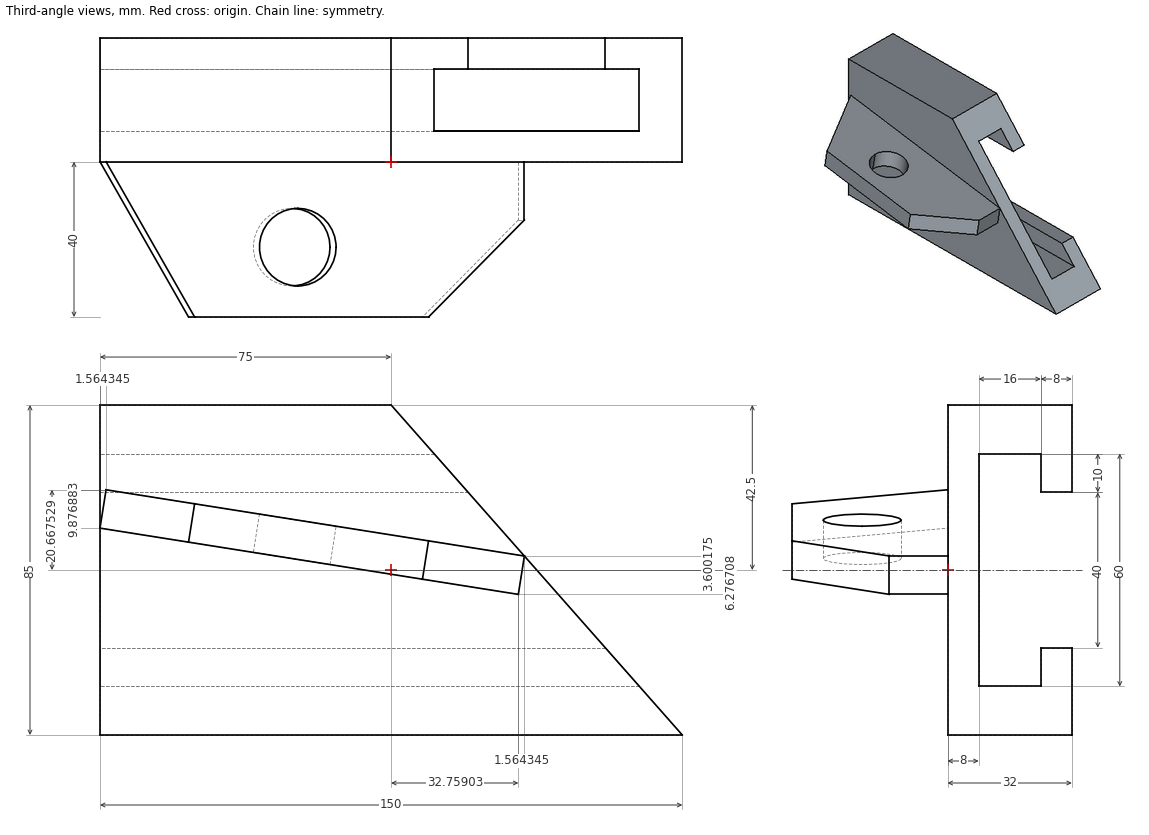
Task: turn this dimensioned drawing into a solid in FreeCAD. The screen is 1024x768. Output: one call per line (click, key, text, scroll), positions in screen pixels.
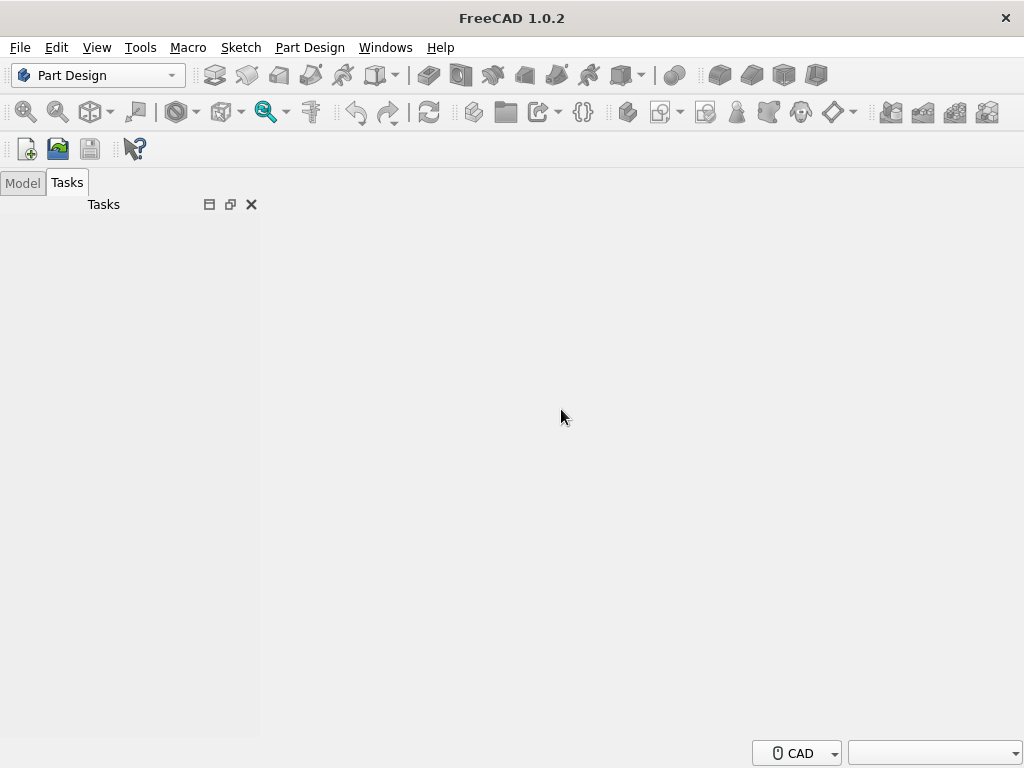
key(ctrl+n)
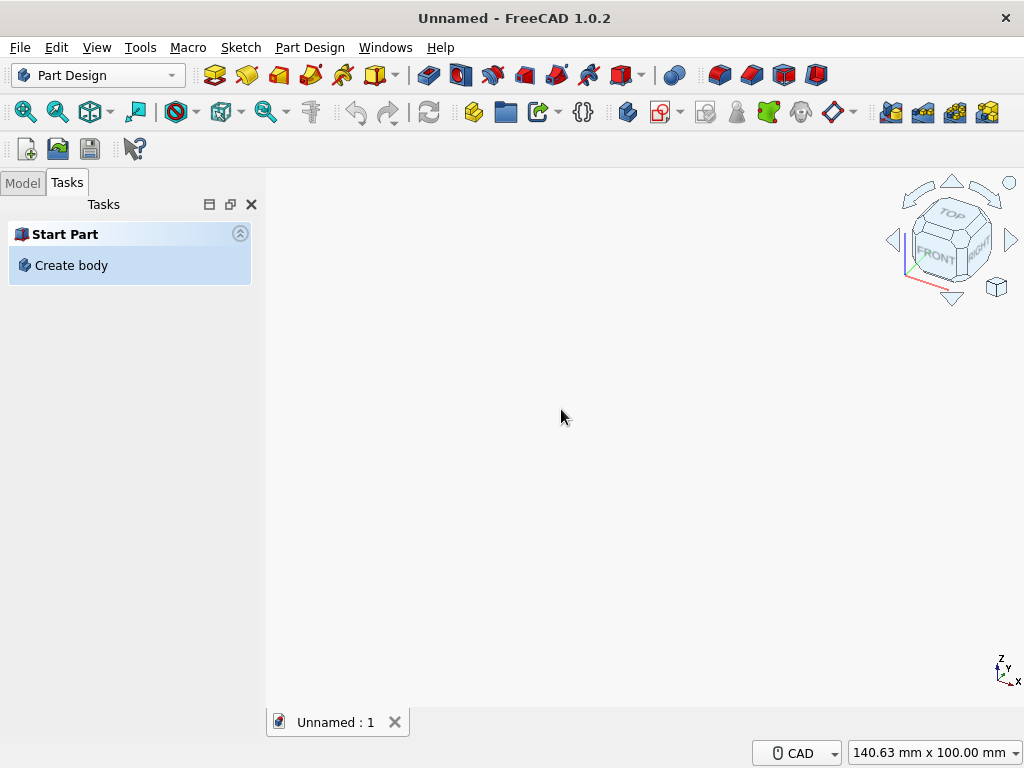
click(660, 112)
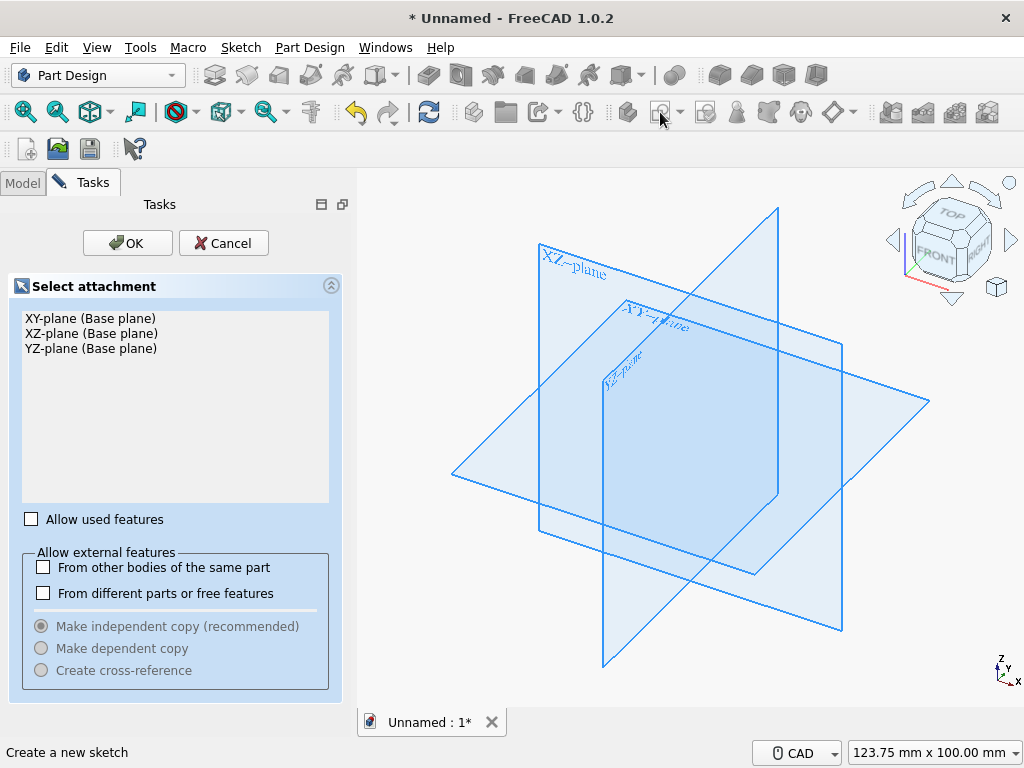
click(82, 334)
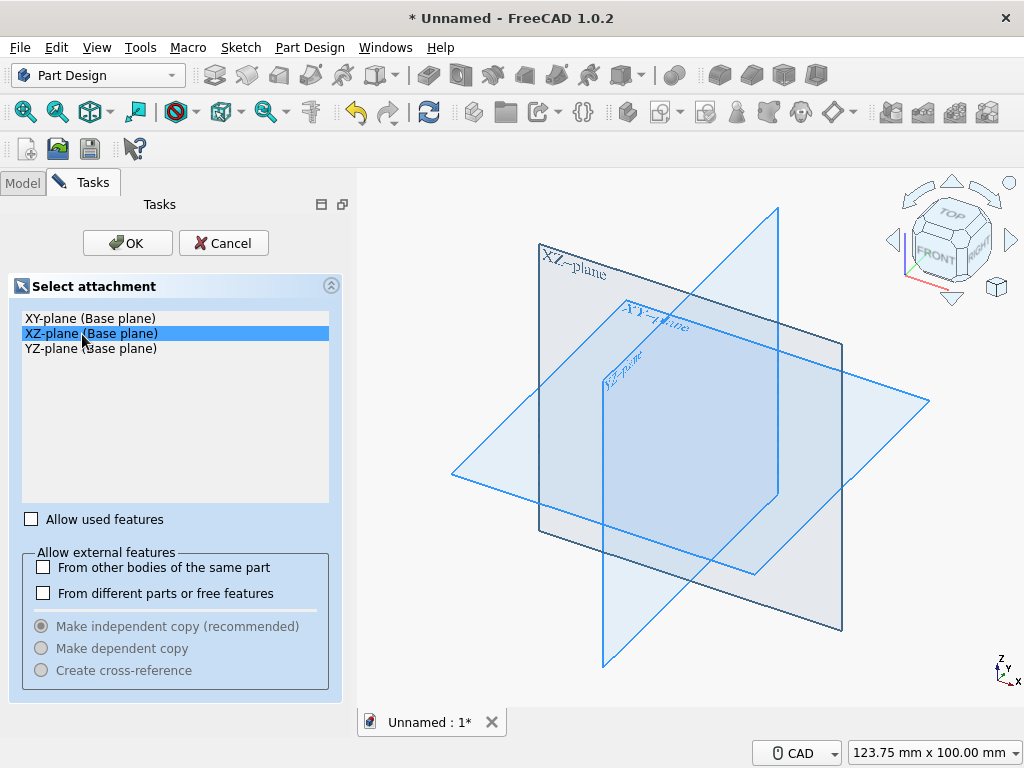
click(128, 243)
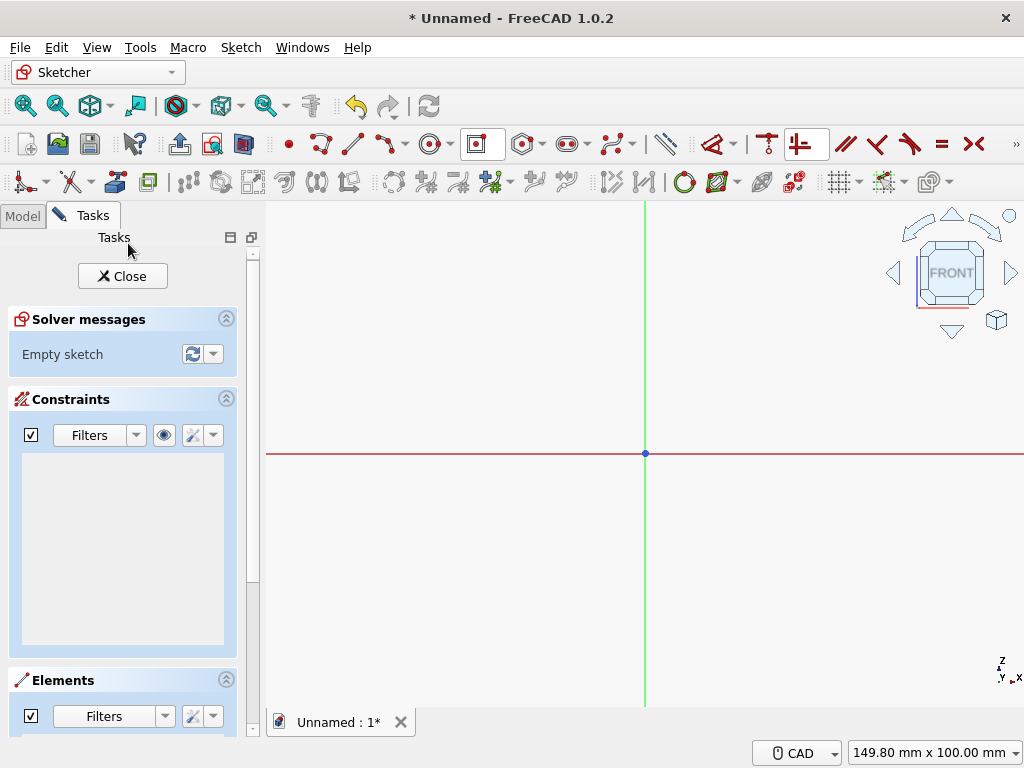
scroll(493, 454, down, 3)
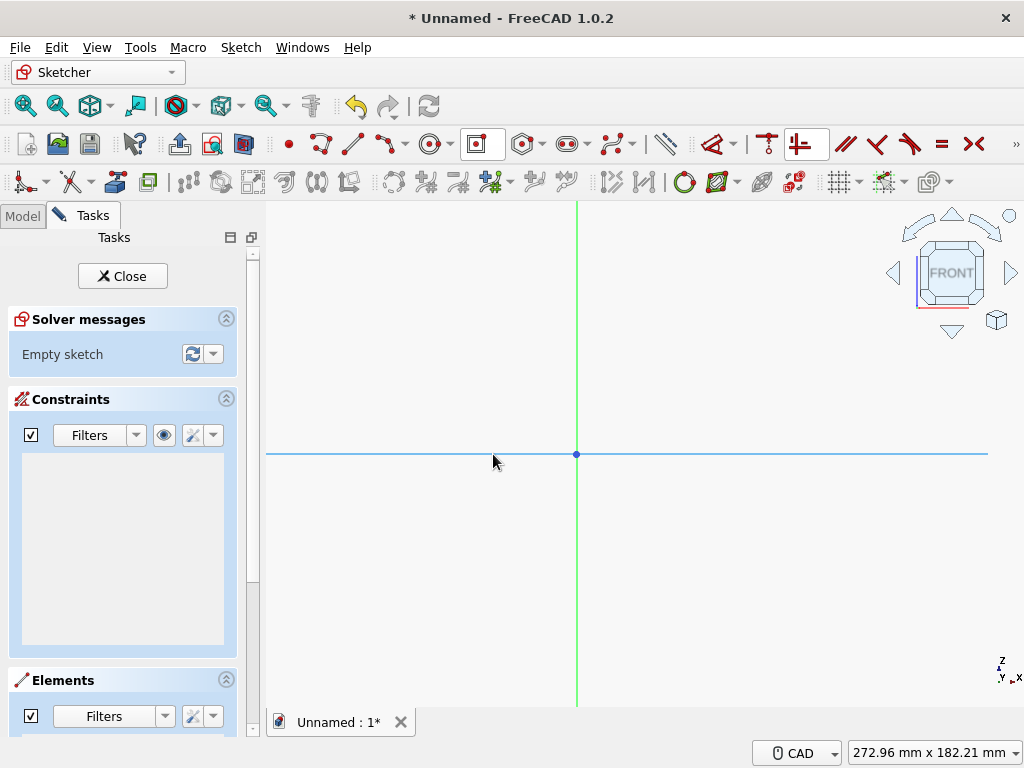
click(322, 144)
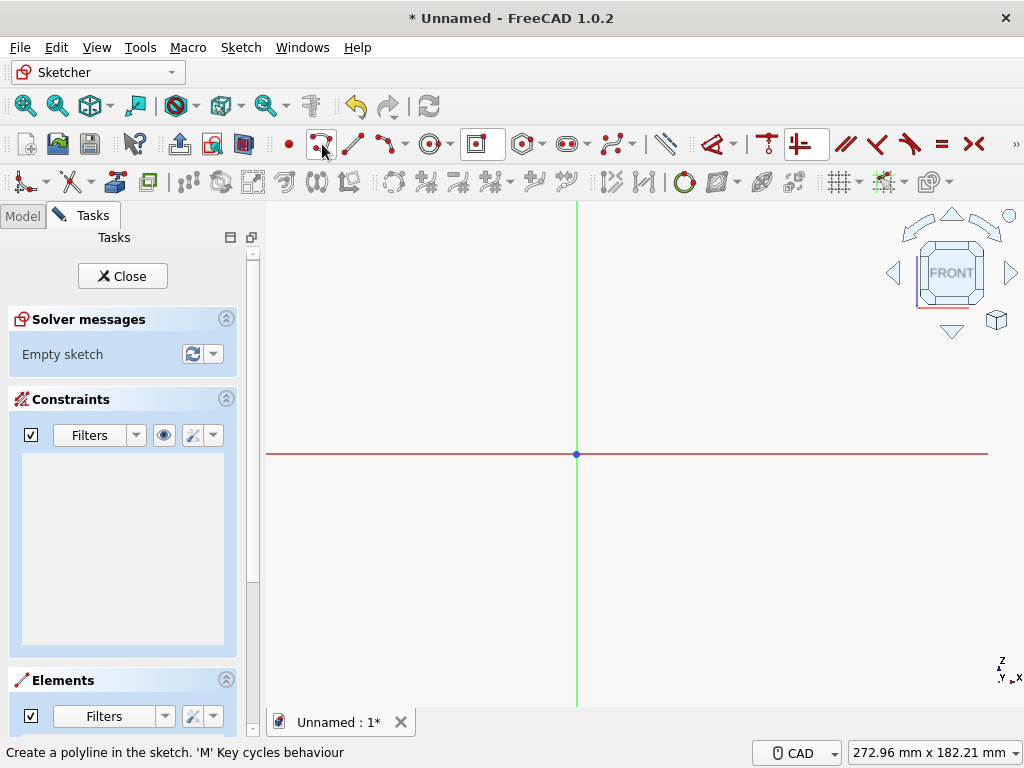
click(577, 336)
click(785, 572)
click(368, 572)
click(368, 336)
click(577, 337)
key(Escape)
key(Escape)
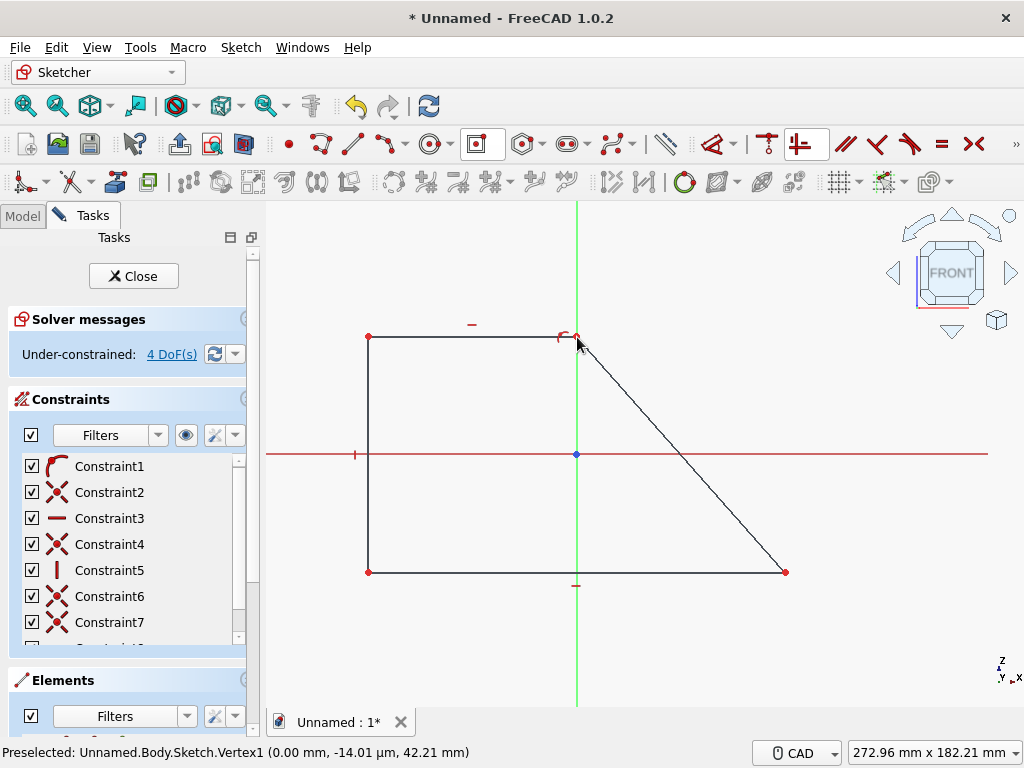
key(d)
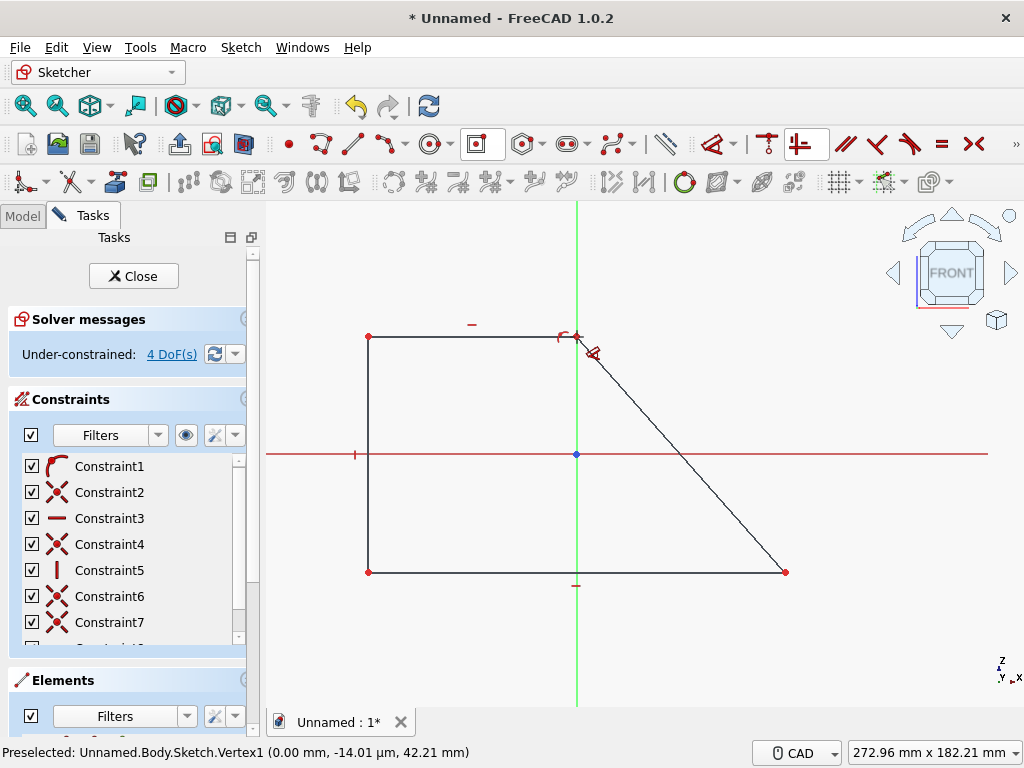
click(368, 502)
click(334, 401)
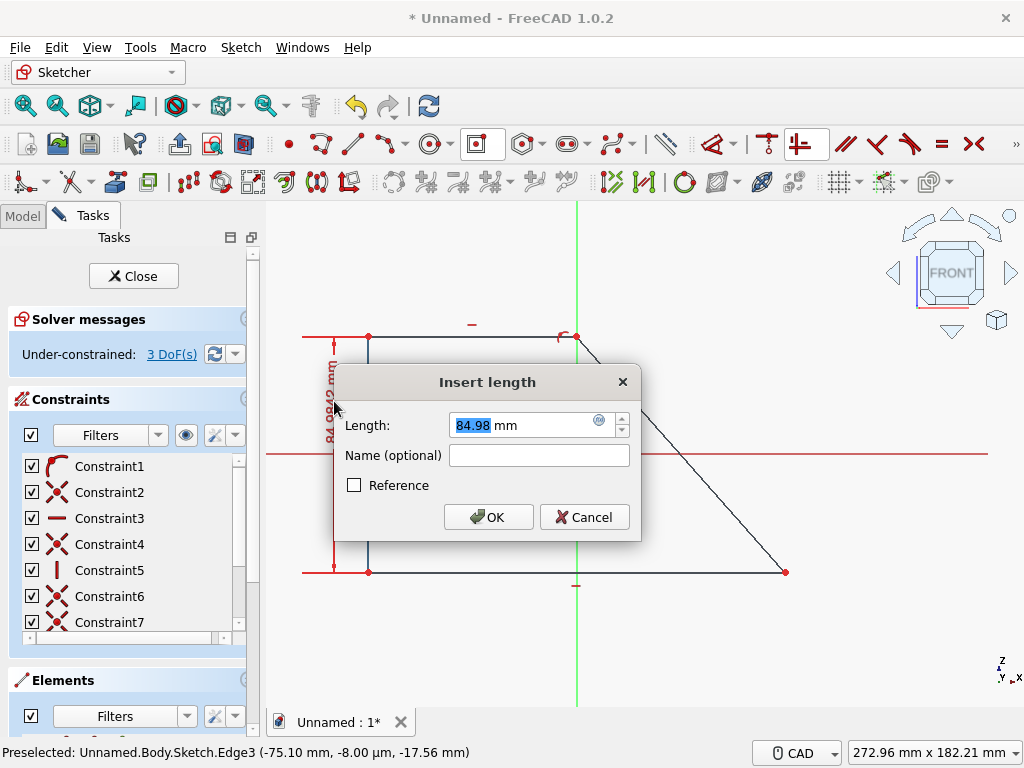
text(85)
key(Return)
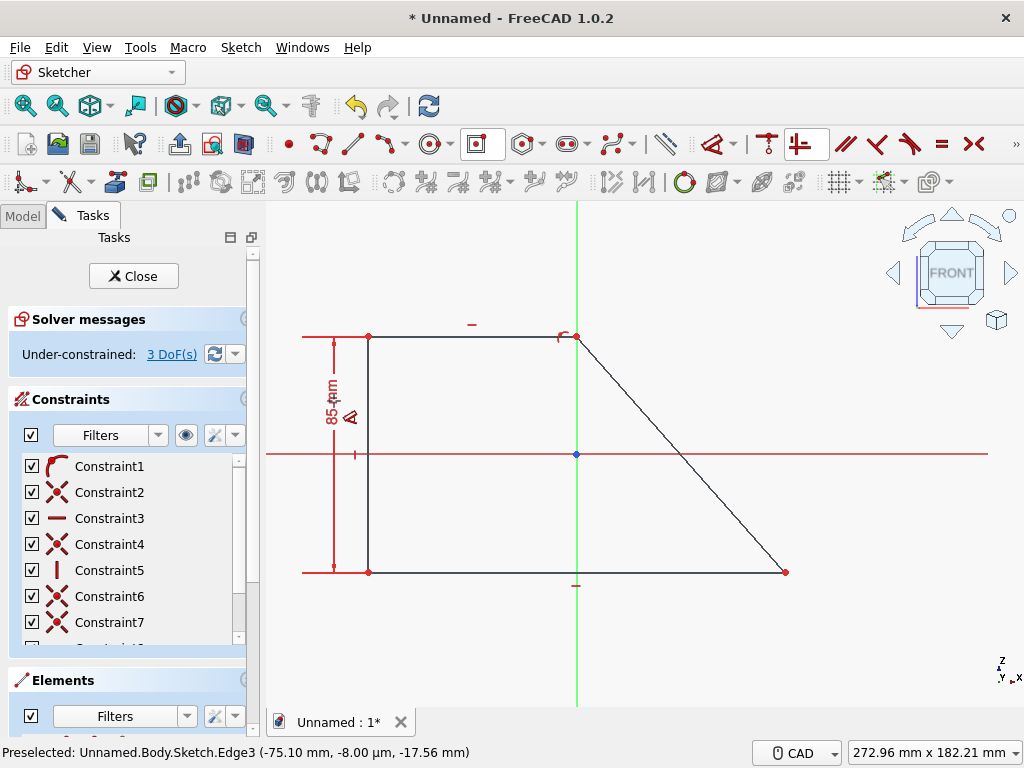
click(431, 337)
click(472, 303)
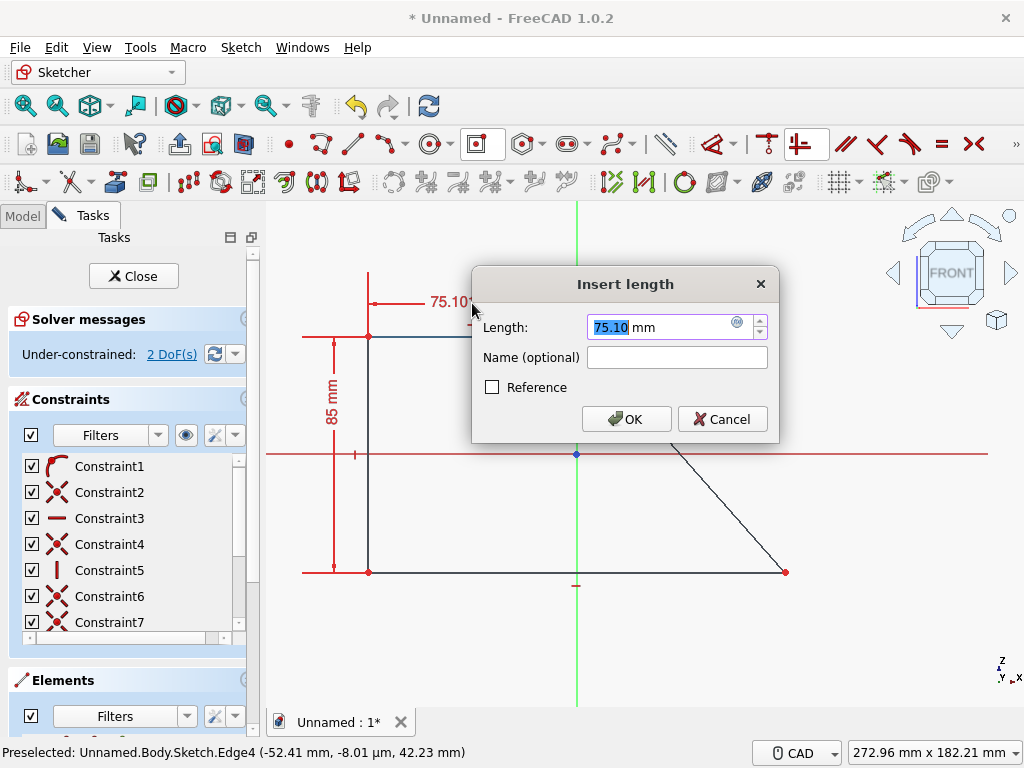
text(75)
key(Return)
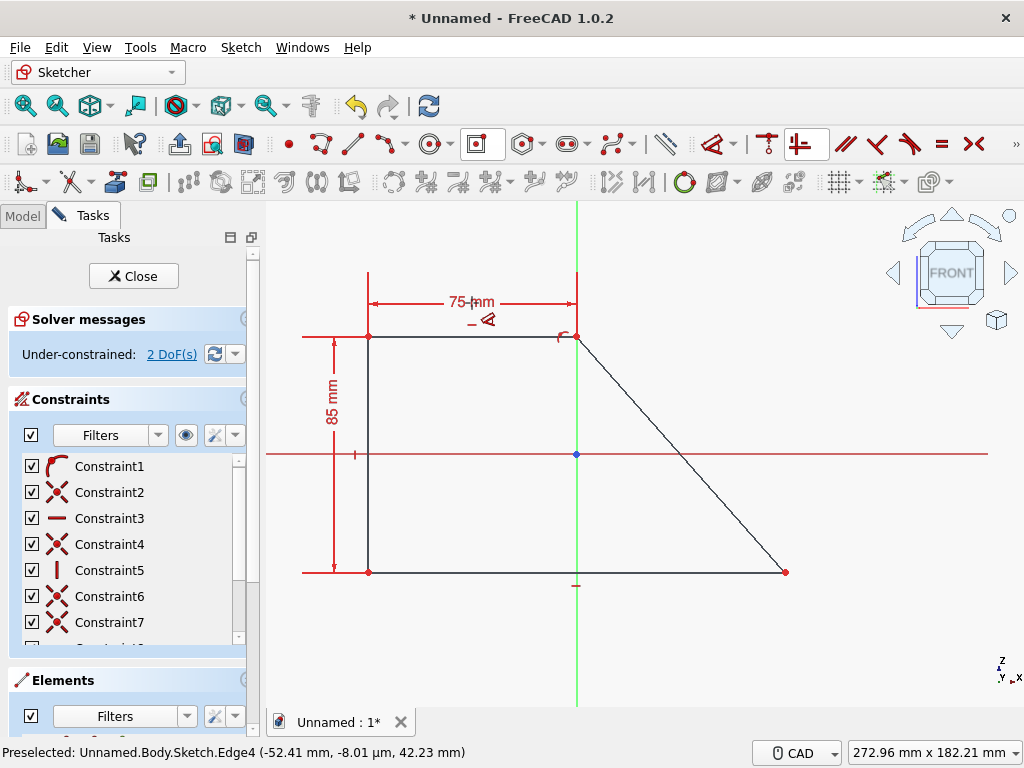
click(660, 573)
click(481, 607)